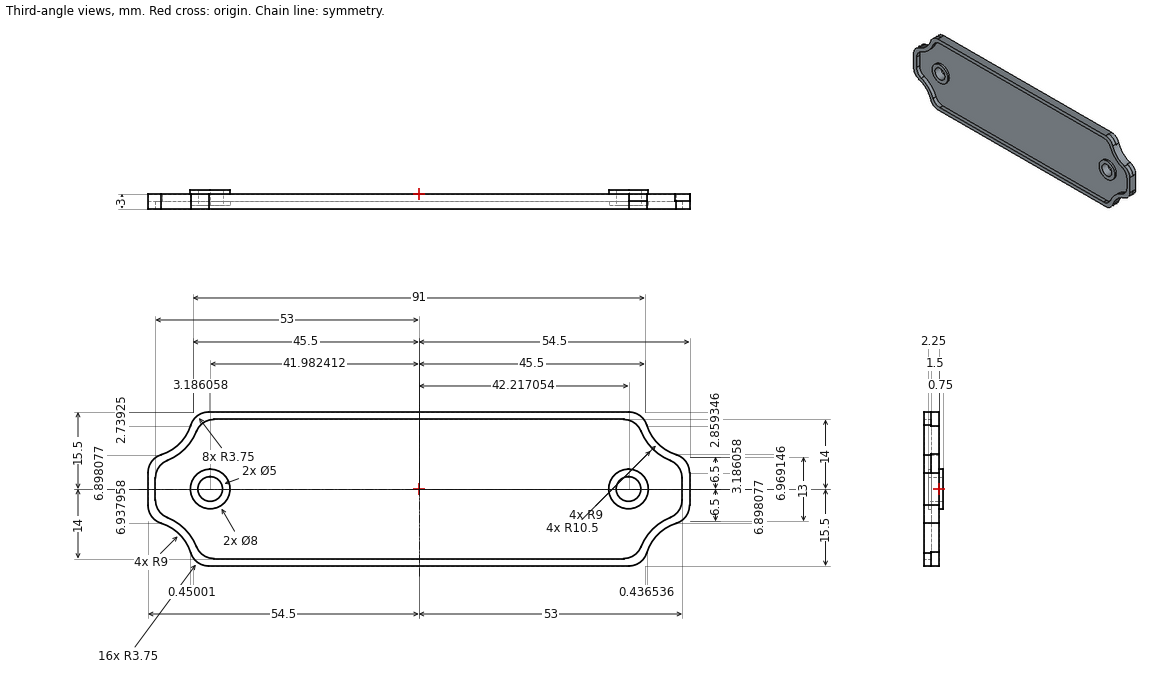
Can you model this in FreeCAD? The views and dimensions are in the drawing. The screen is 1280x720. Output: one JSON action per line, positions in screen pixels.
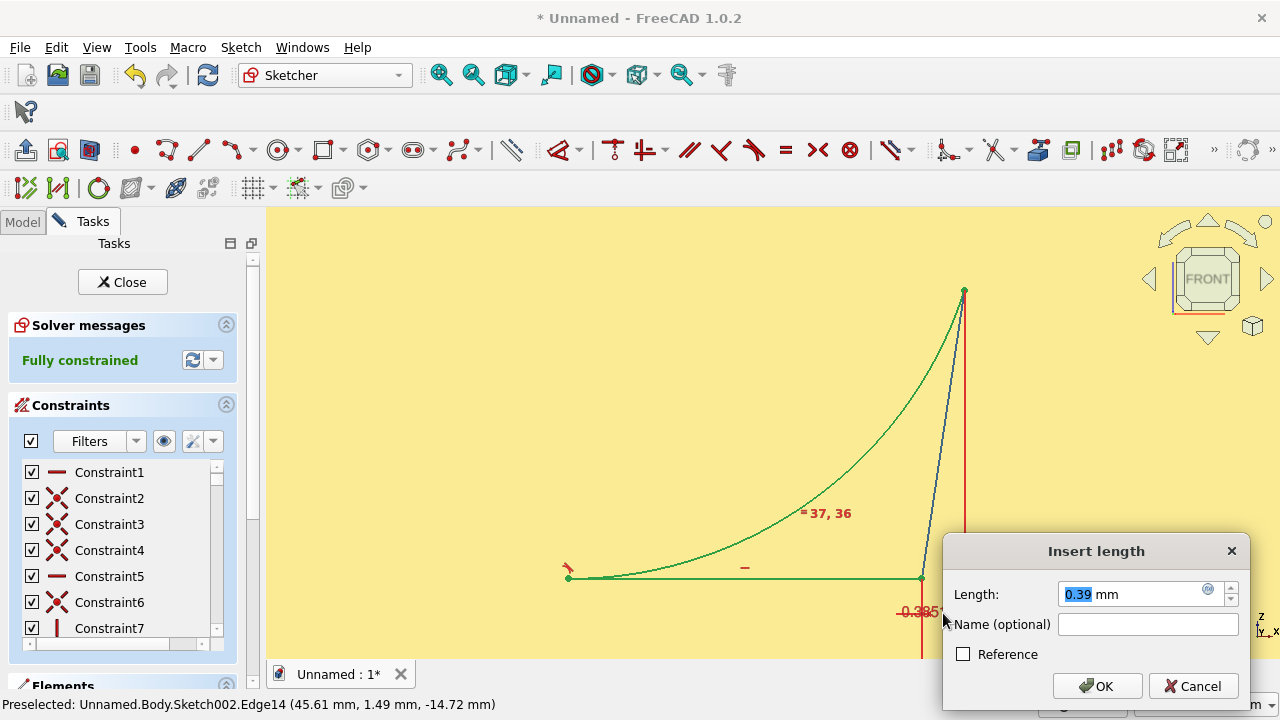
{"action": "type", "text": "0.436536"}
{"action": "key", "text": "Return"}
{"action": "key", "text": "Escape"}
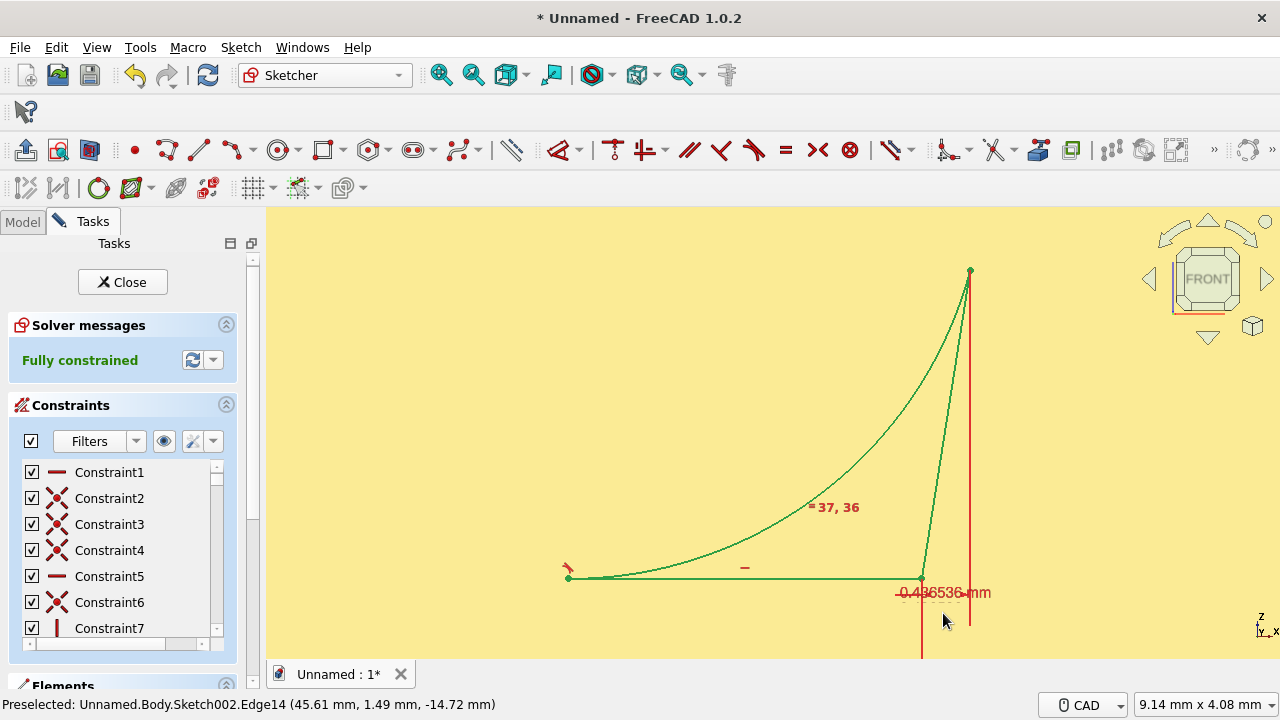
{"action": "left_click", "coordinate": [123, 282]}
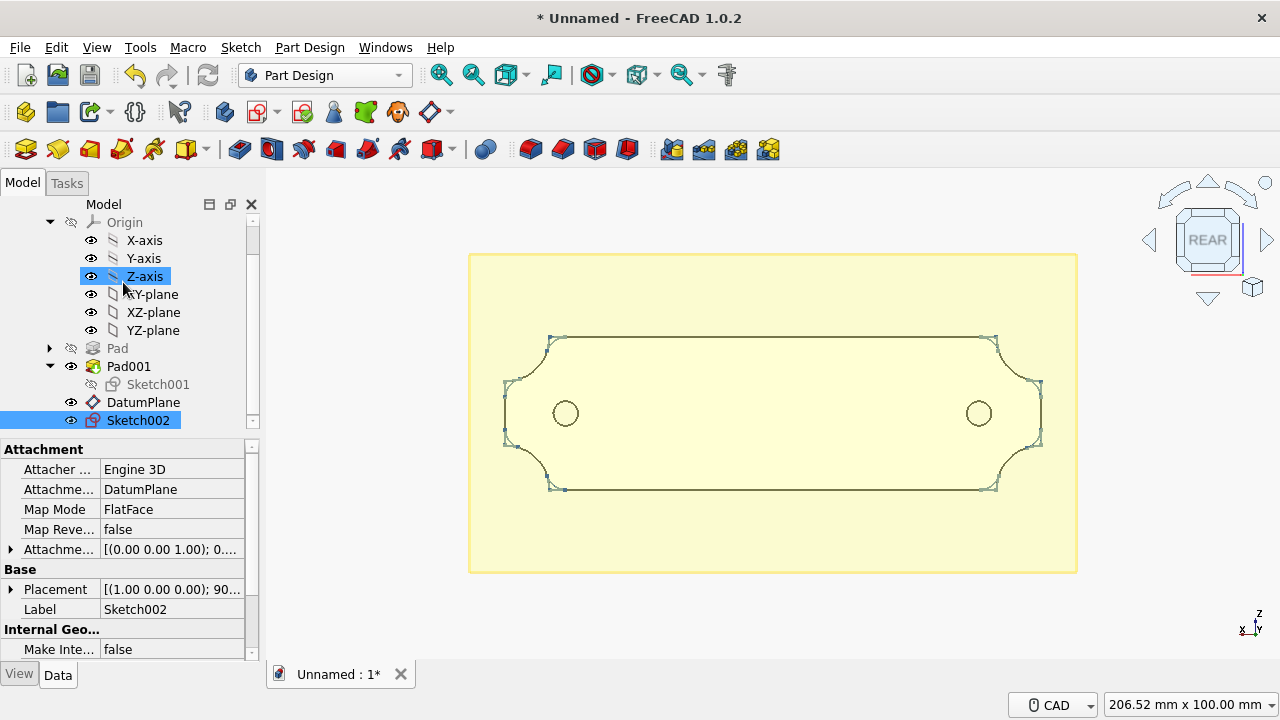
{"action": "left_click", "coordinate": [240, 150]}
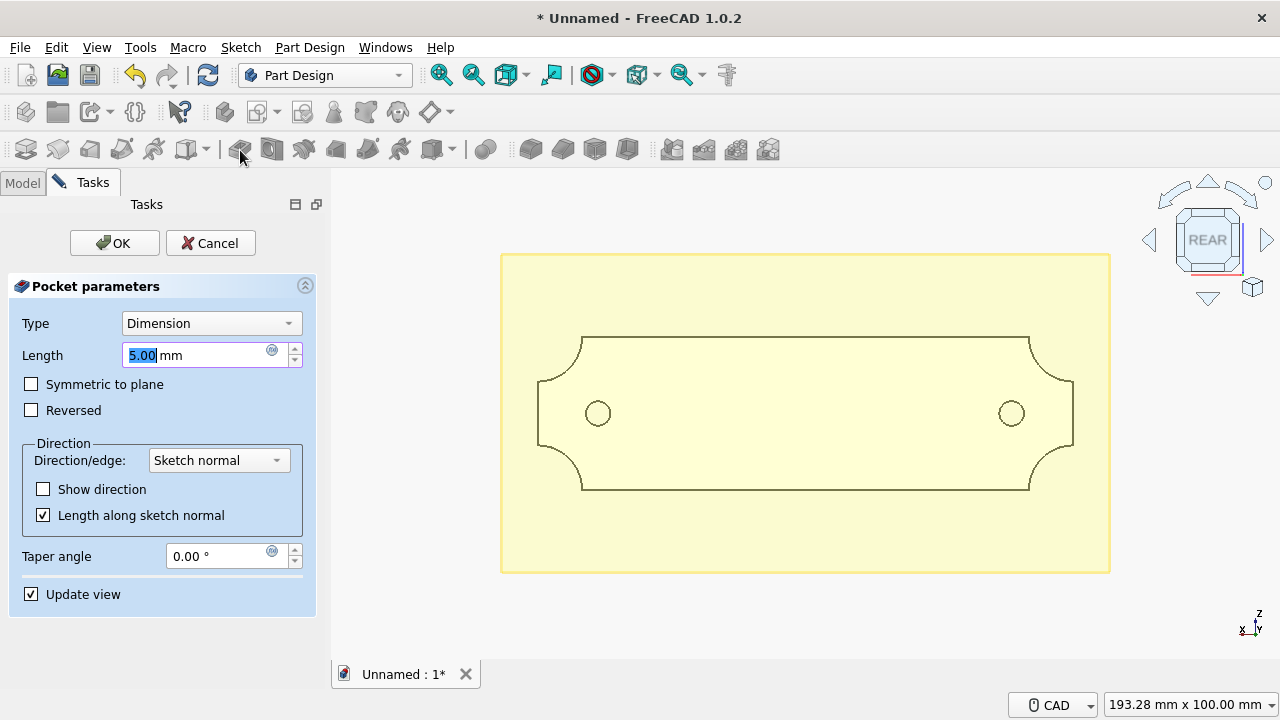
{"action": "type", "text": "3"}
{"action": "key", "text": "Tab"}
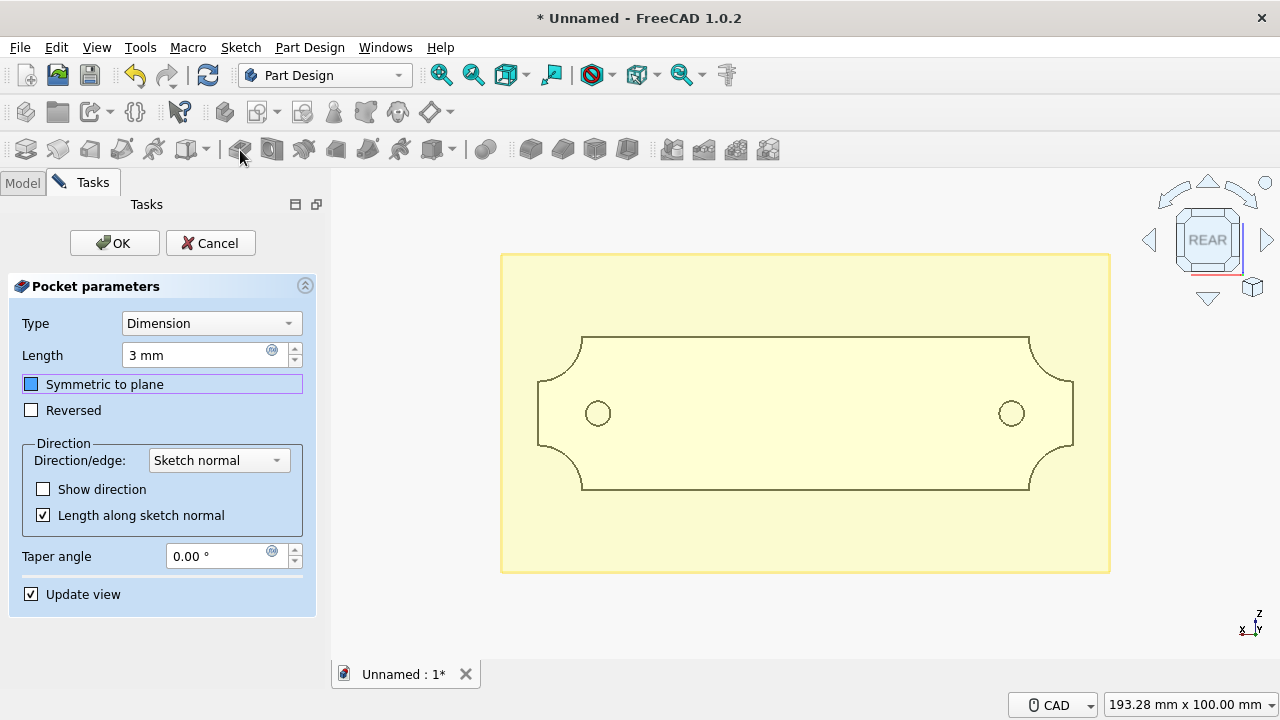
{"action": "left_click", "coordinate": [30, 410]}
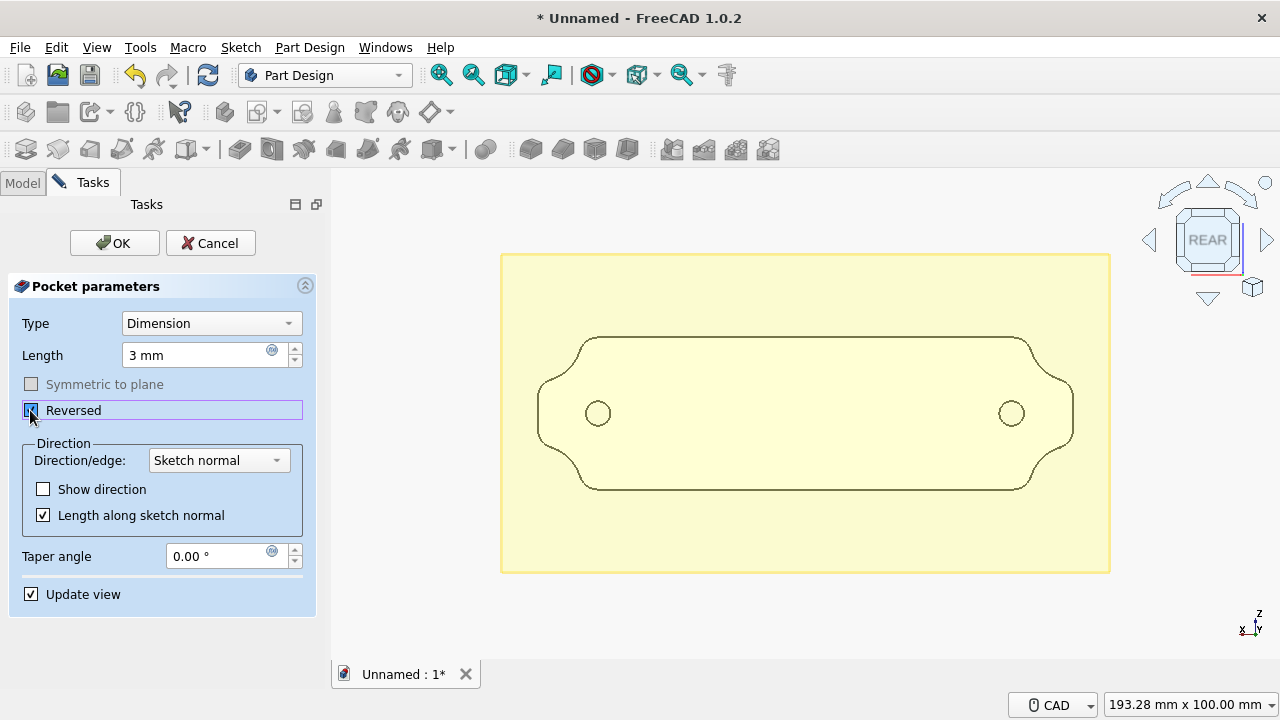
{"action": "left_click", "coordinate": [115, 243]}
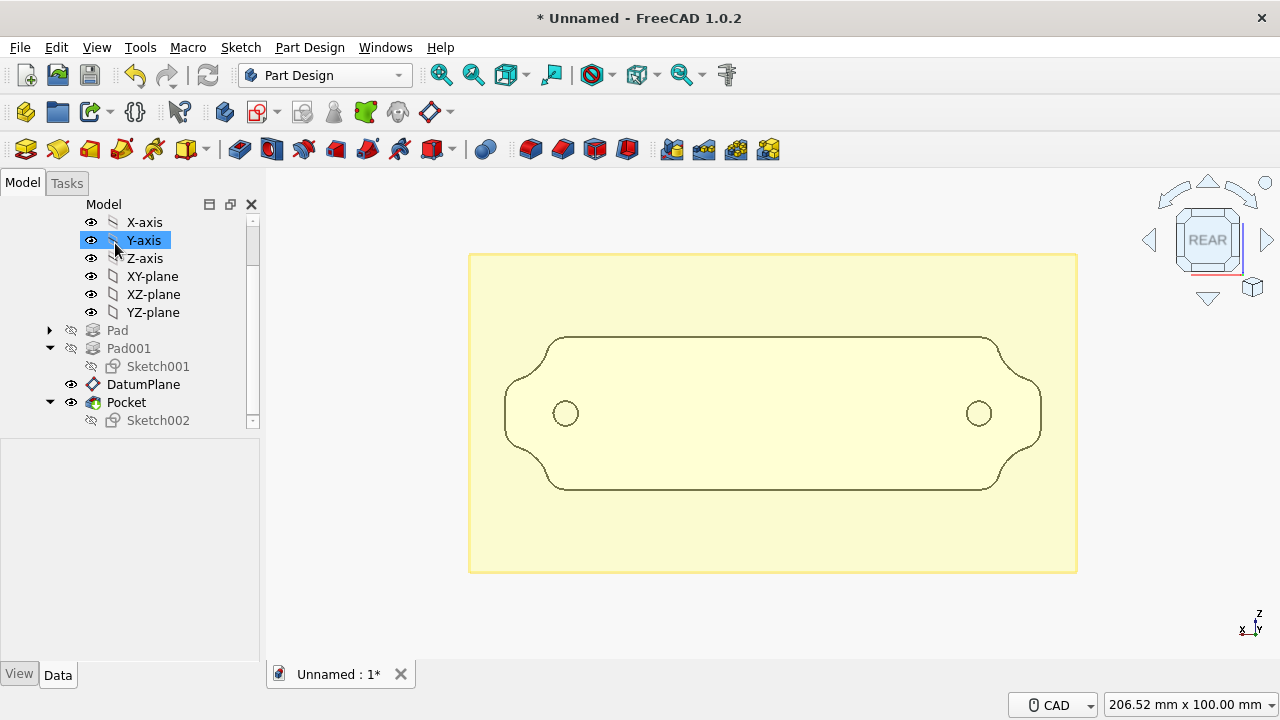
{"action": "left_click", "coordinate": [116, 384]}
{"action": "key", "text": "space"}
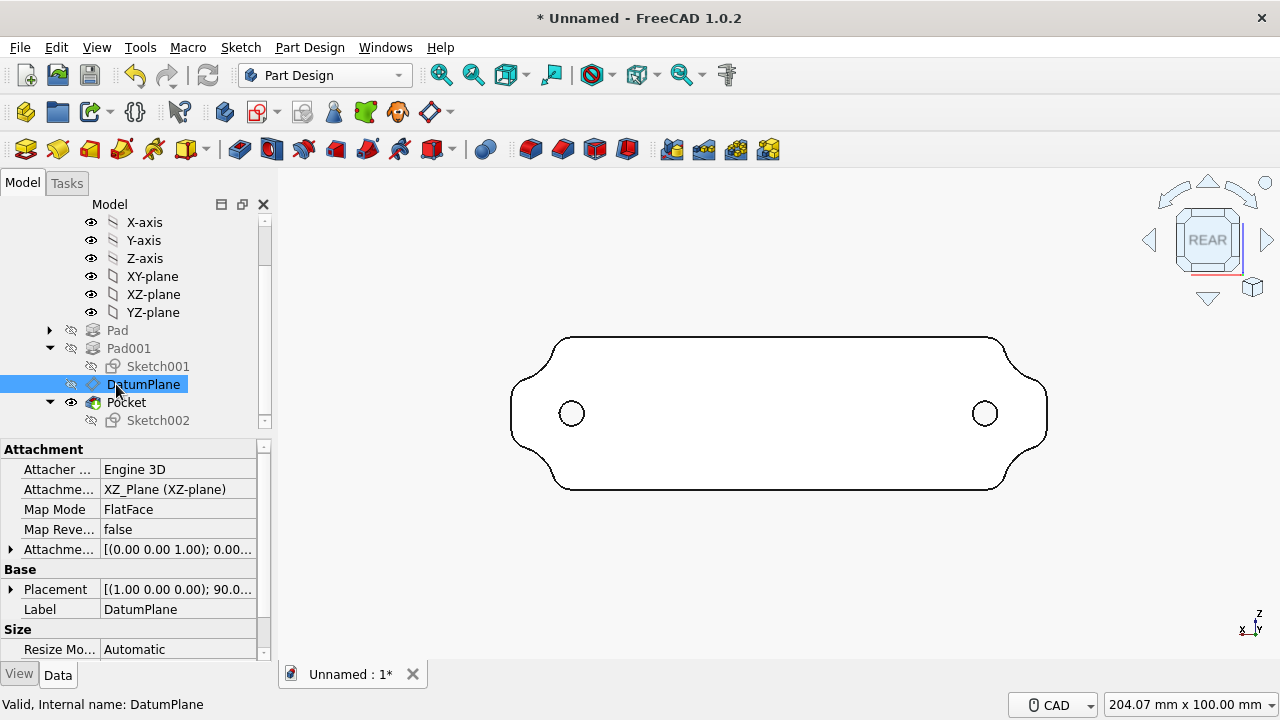
{"action": "left_click", "coordinate": [318, 619]}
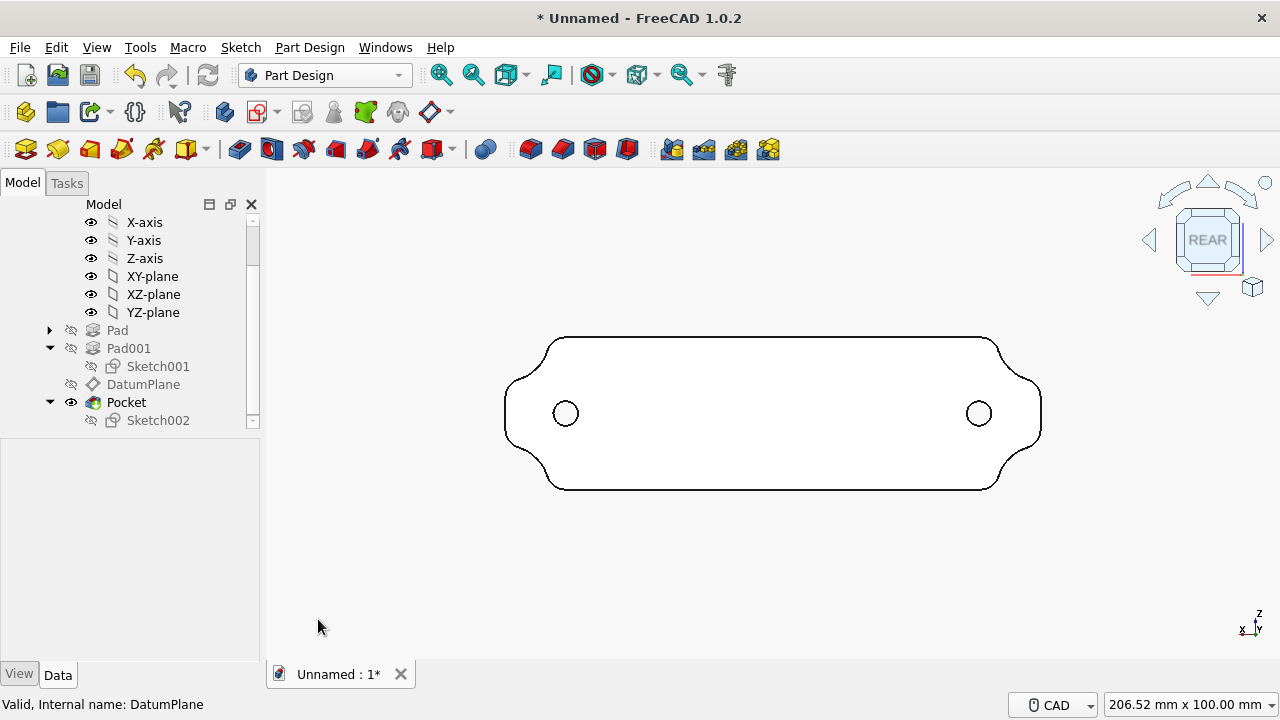
{"action": "left_click", "coordinate": [258, 112]}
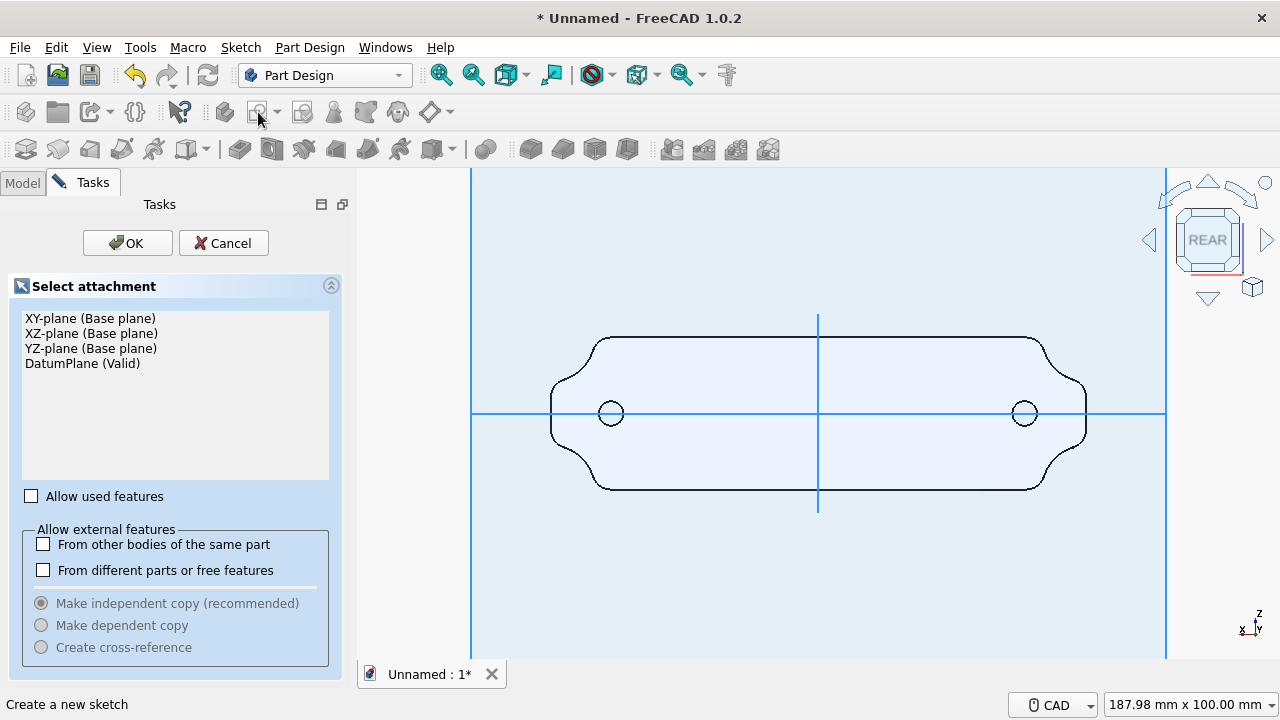
{"action": "left_click", "coordinate": [82, 334]}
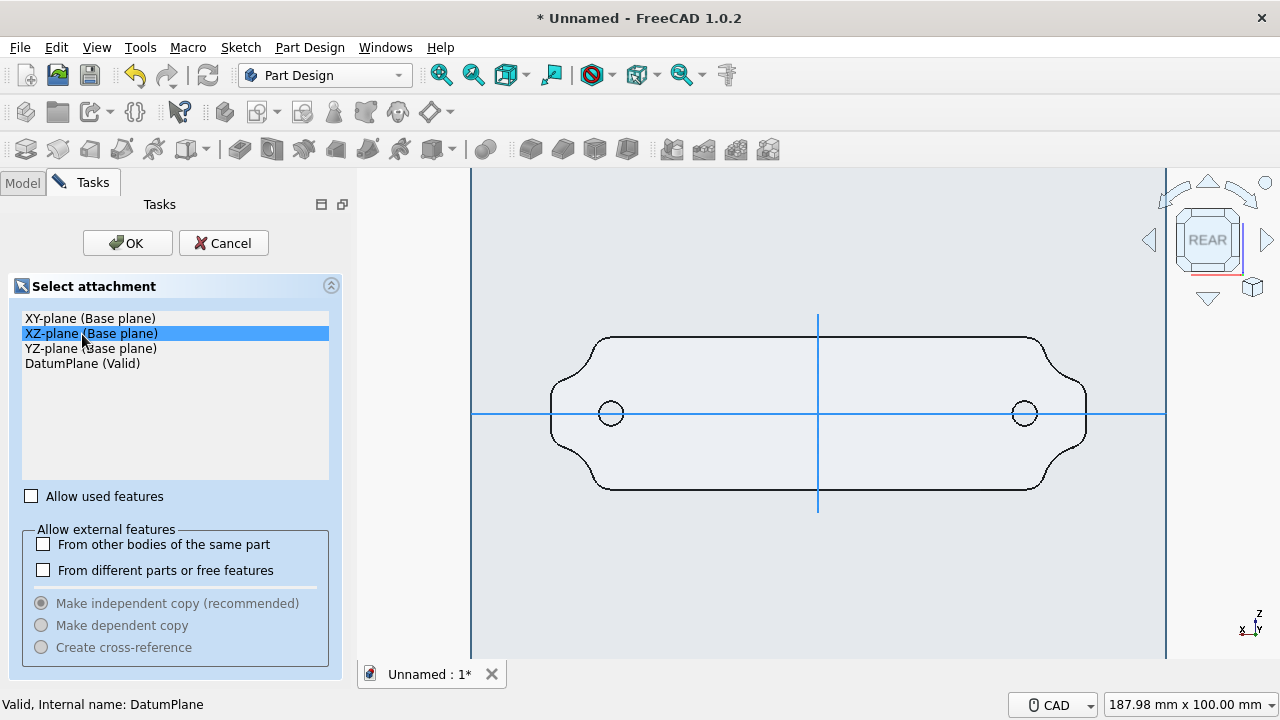
{"action": "left_click", "coordinate": [128, 243]}